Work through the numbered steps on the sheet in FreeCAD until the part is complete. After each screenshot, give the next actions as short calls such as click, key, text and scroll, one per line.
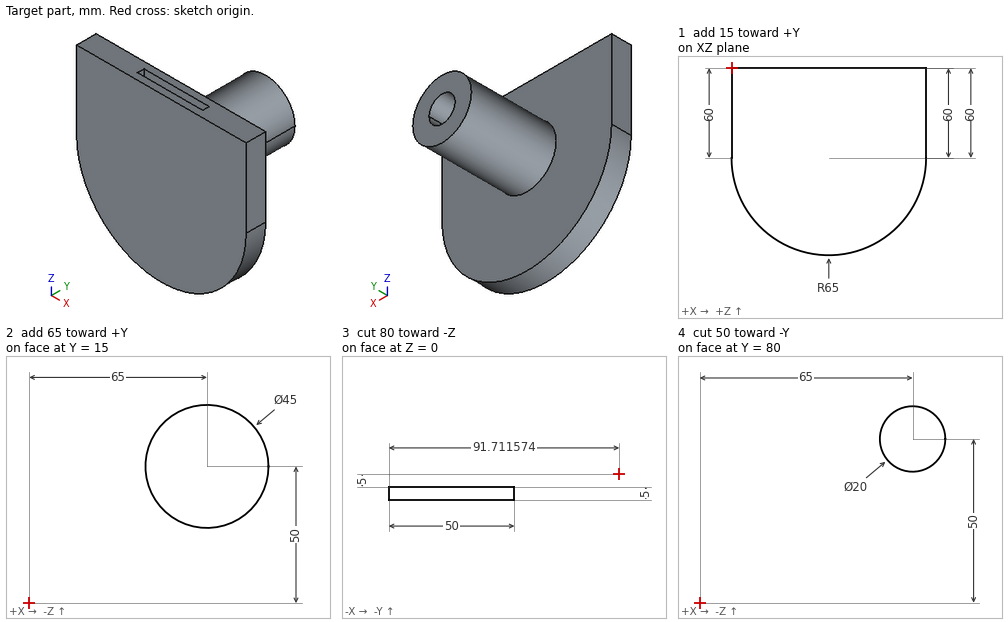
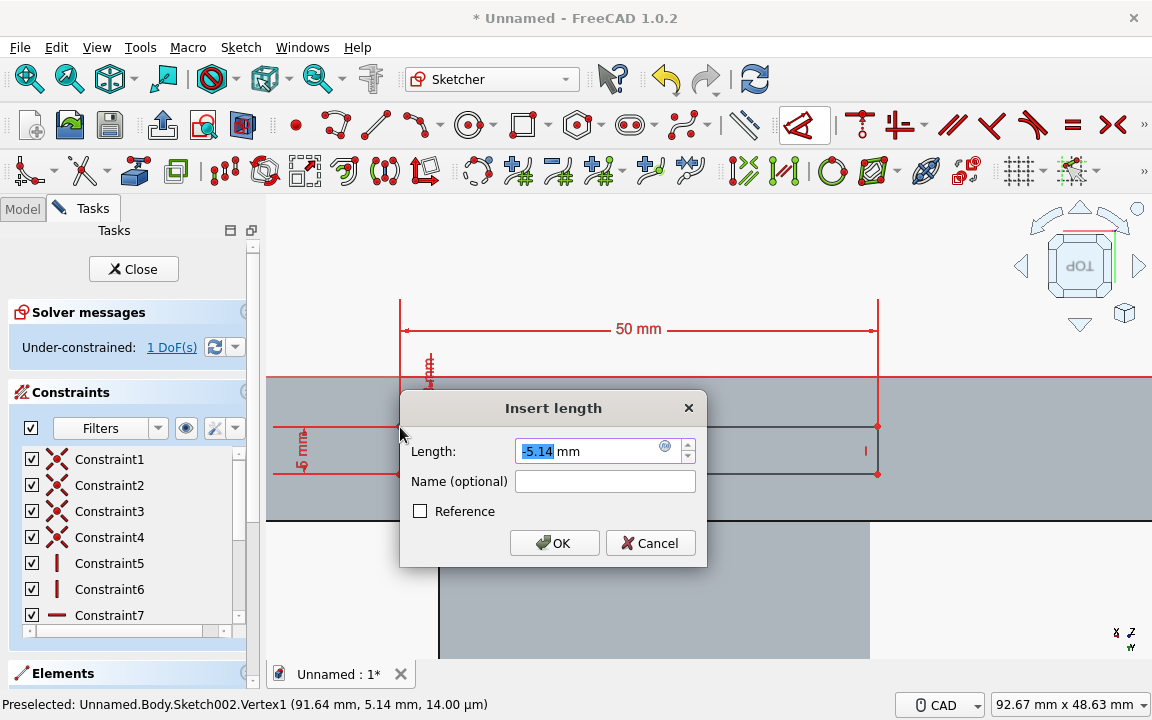
text(-5)
key(Return)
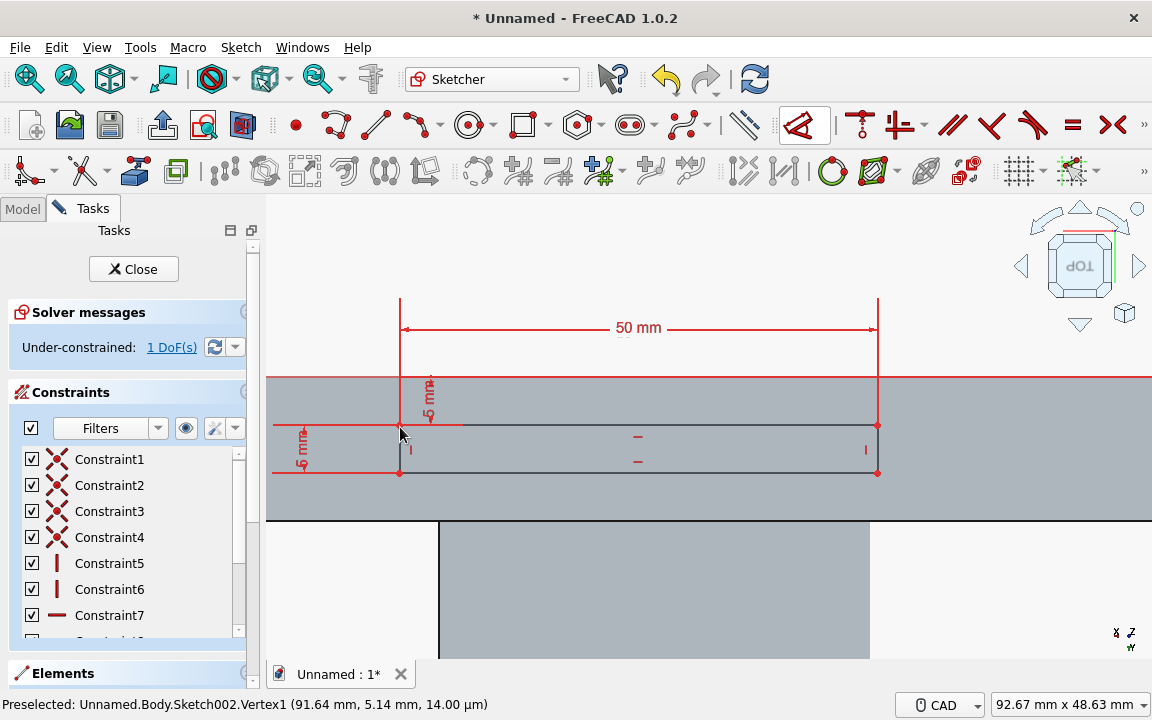
click(400, 425)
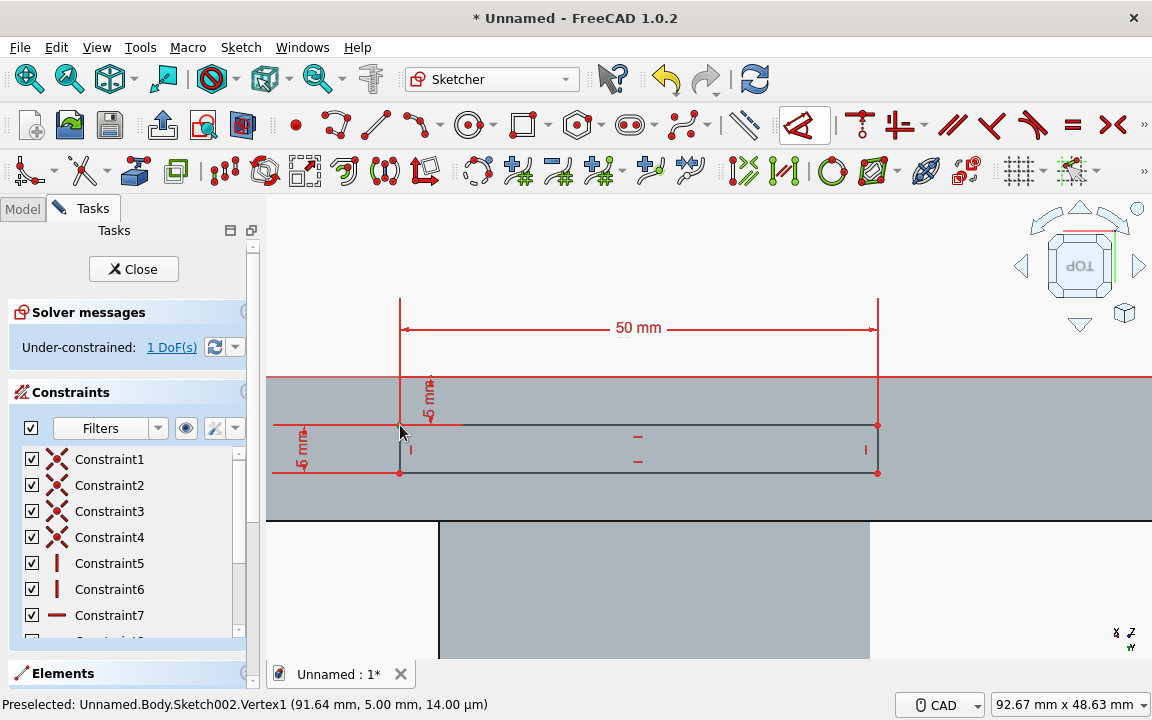
click(824, 126)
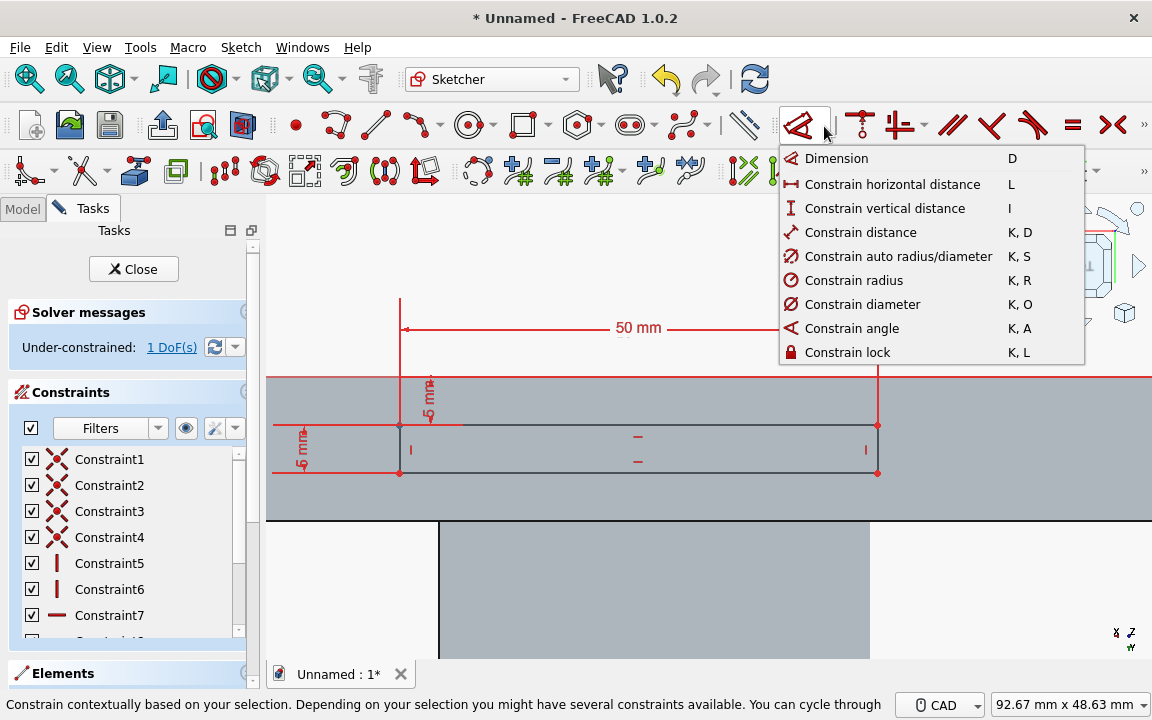
click(932, 184)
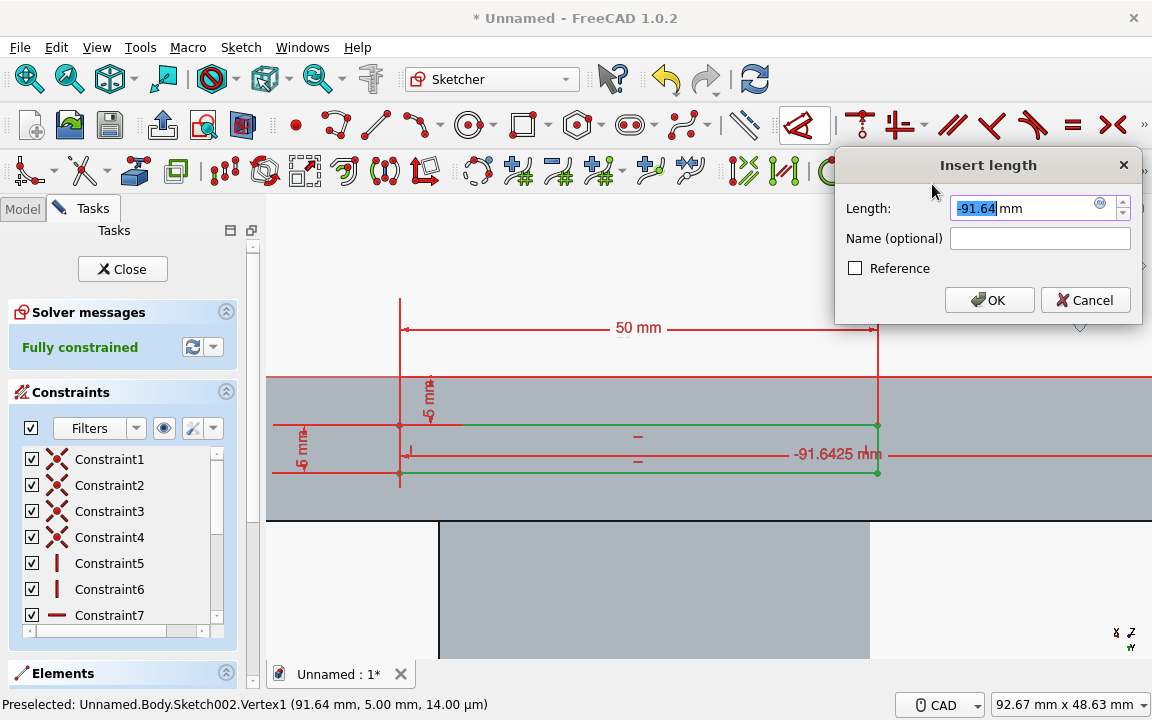
text(-91.711574)
key(Return)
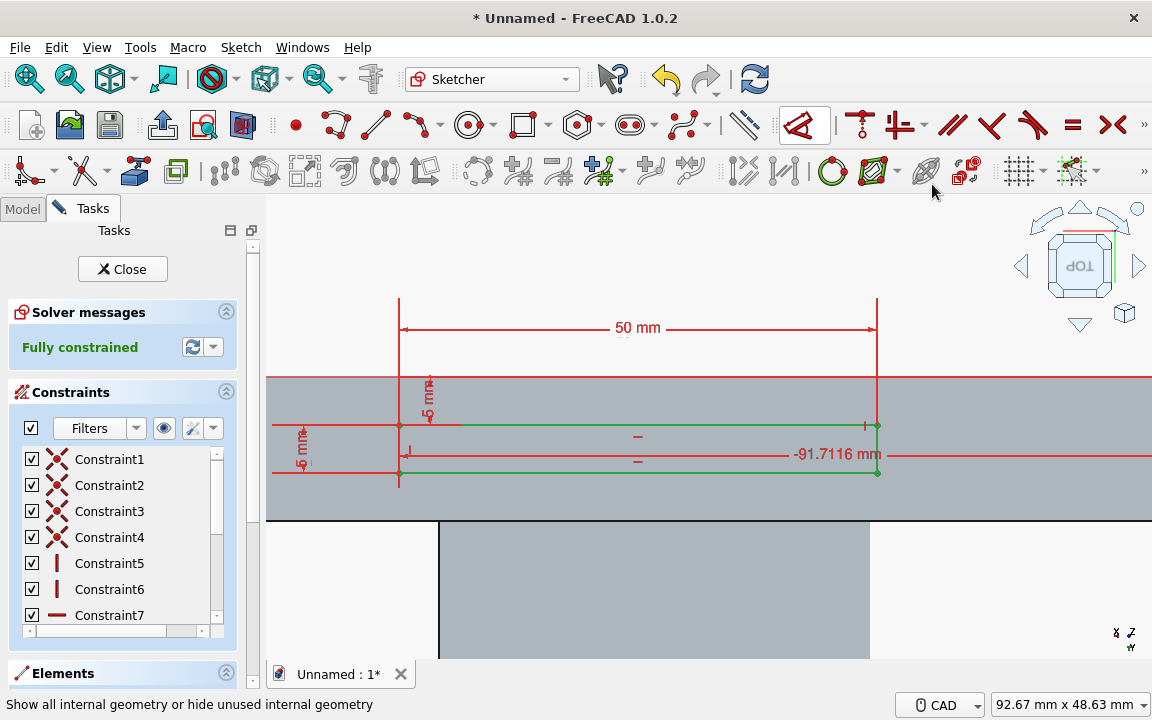
click(123, 269)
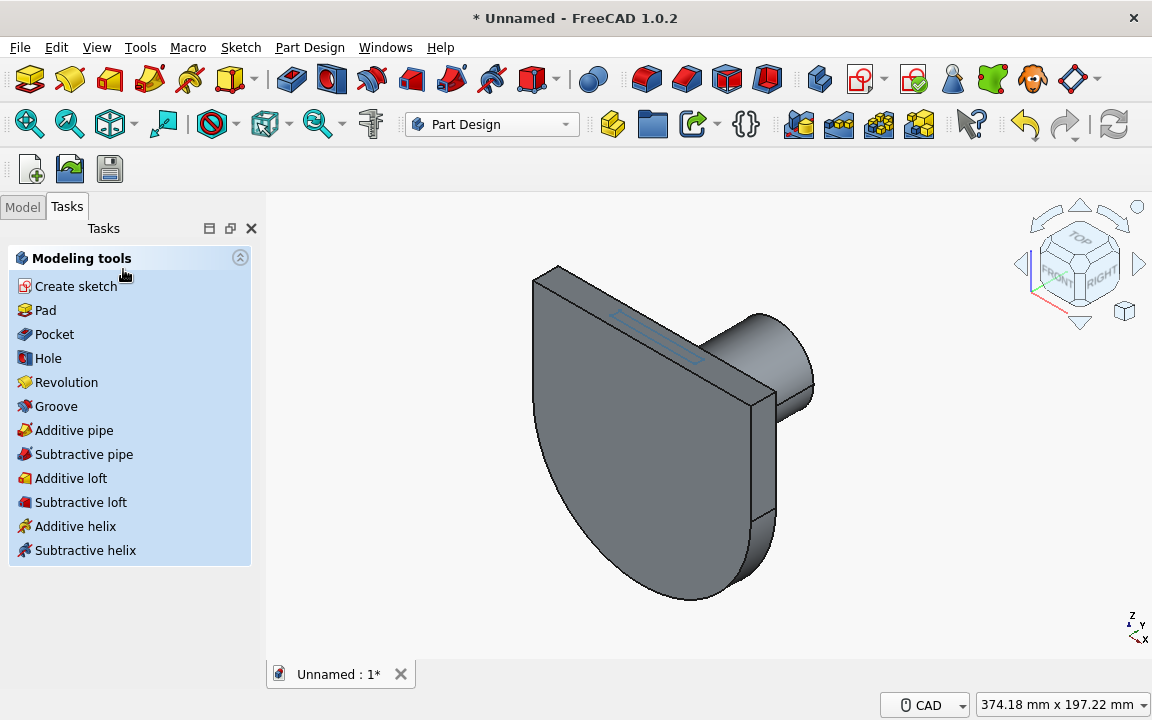
click(292, 80)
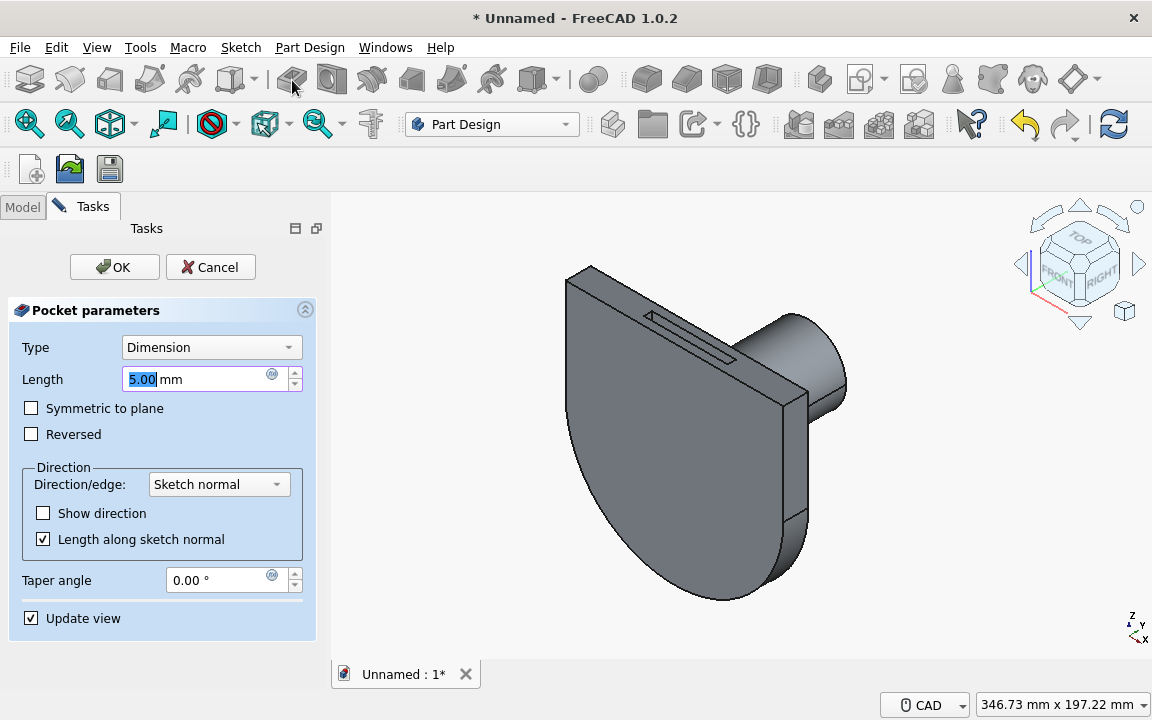
text(80)
key(Tab)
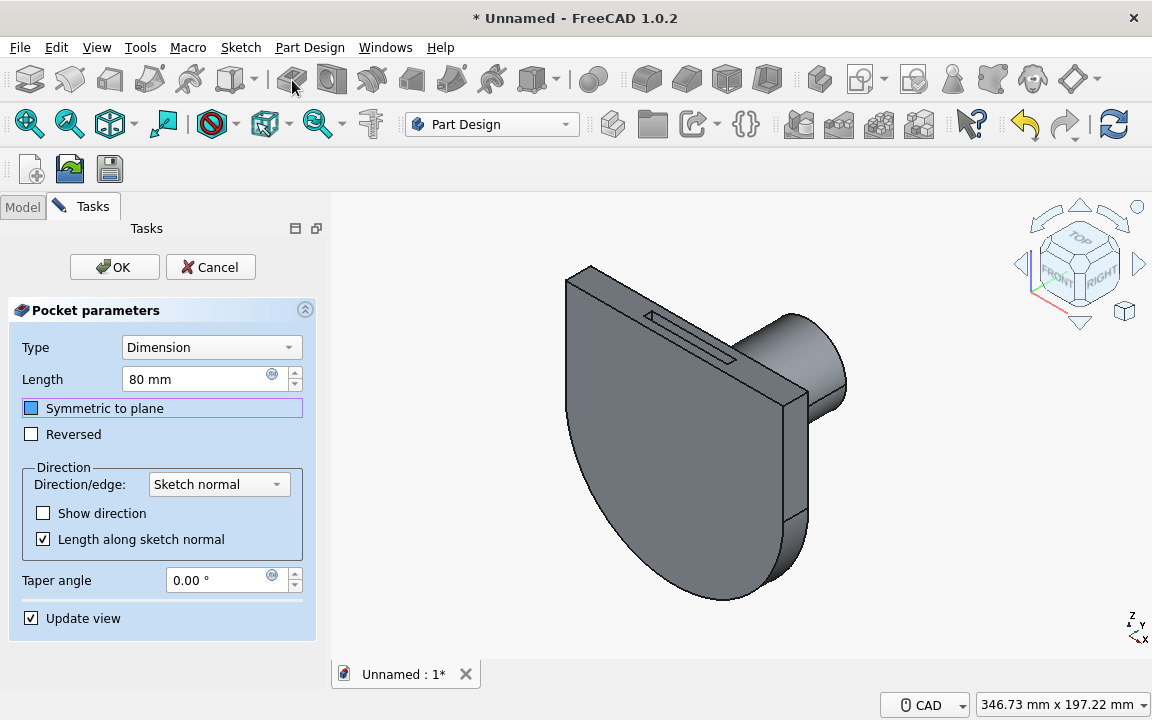
click(115, 267)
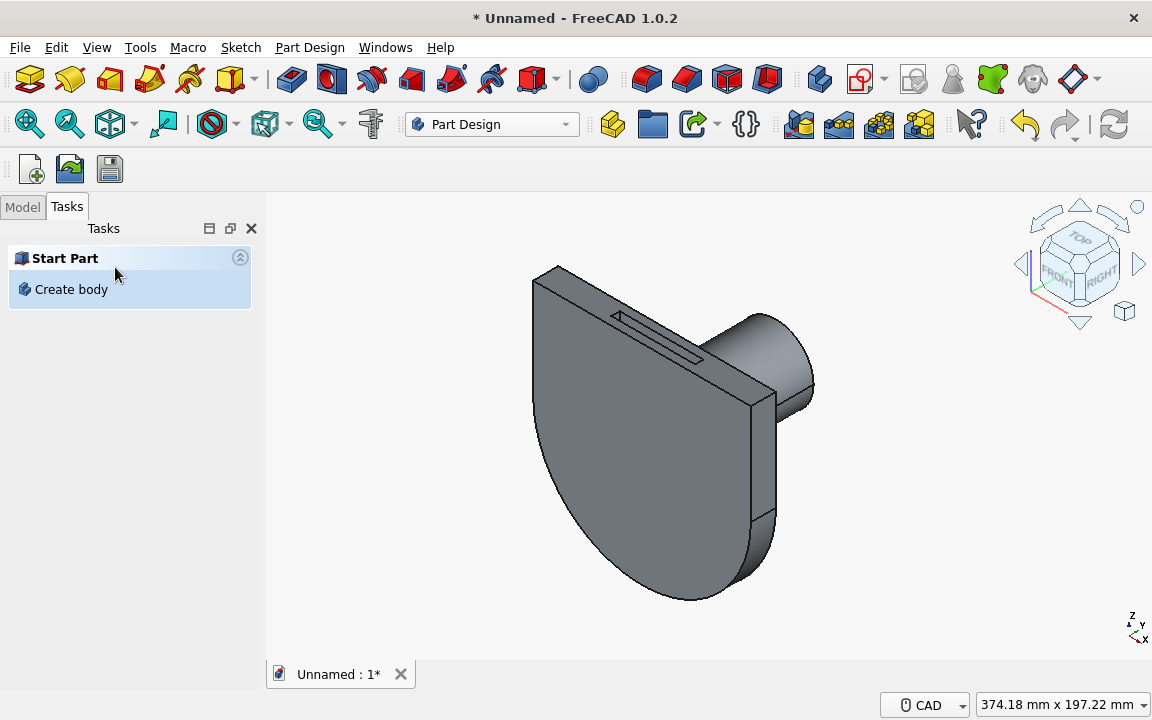
key(4)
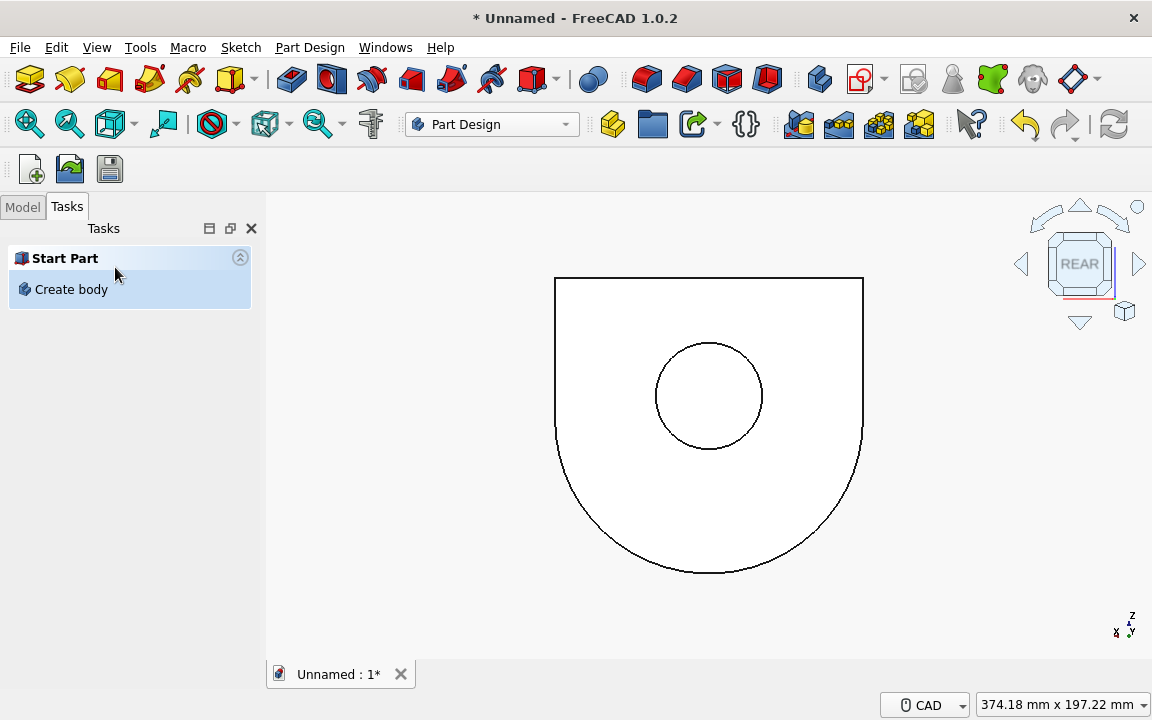
click(709, 395)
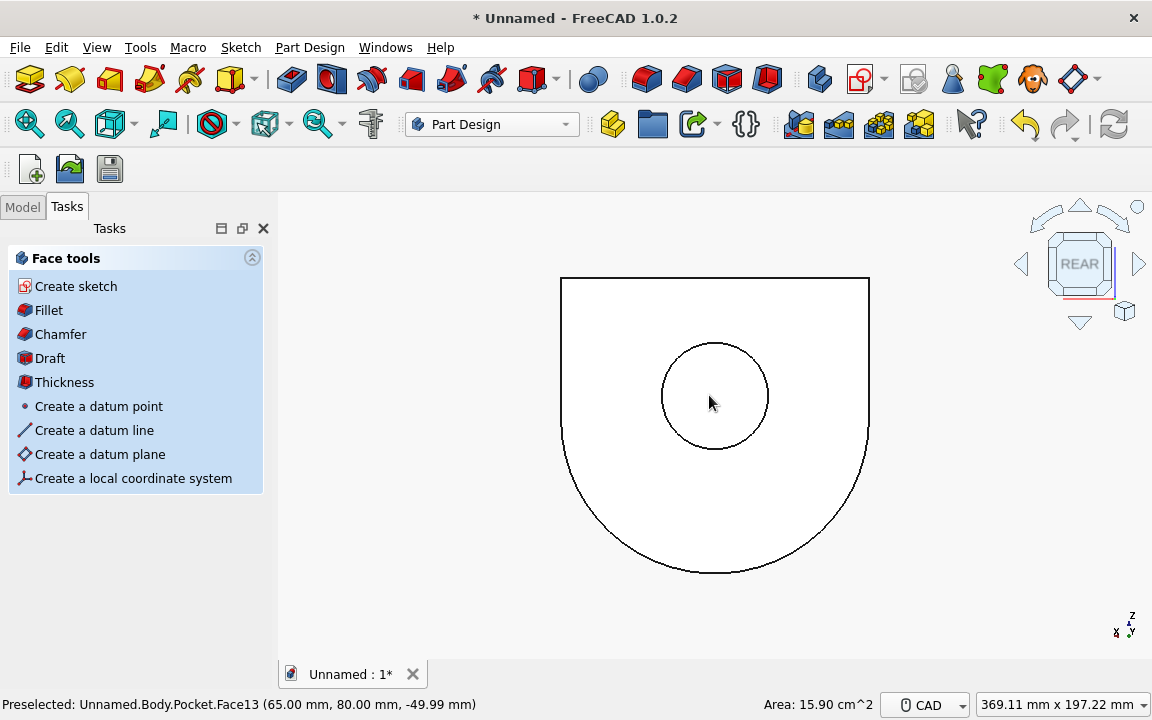
click(860, 80)